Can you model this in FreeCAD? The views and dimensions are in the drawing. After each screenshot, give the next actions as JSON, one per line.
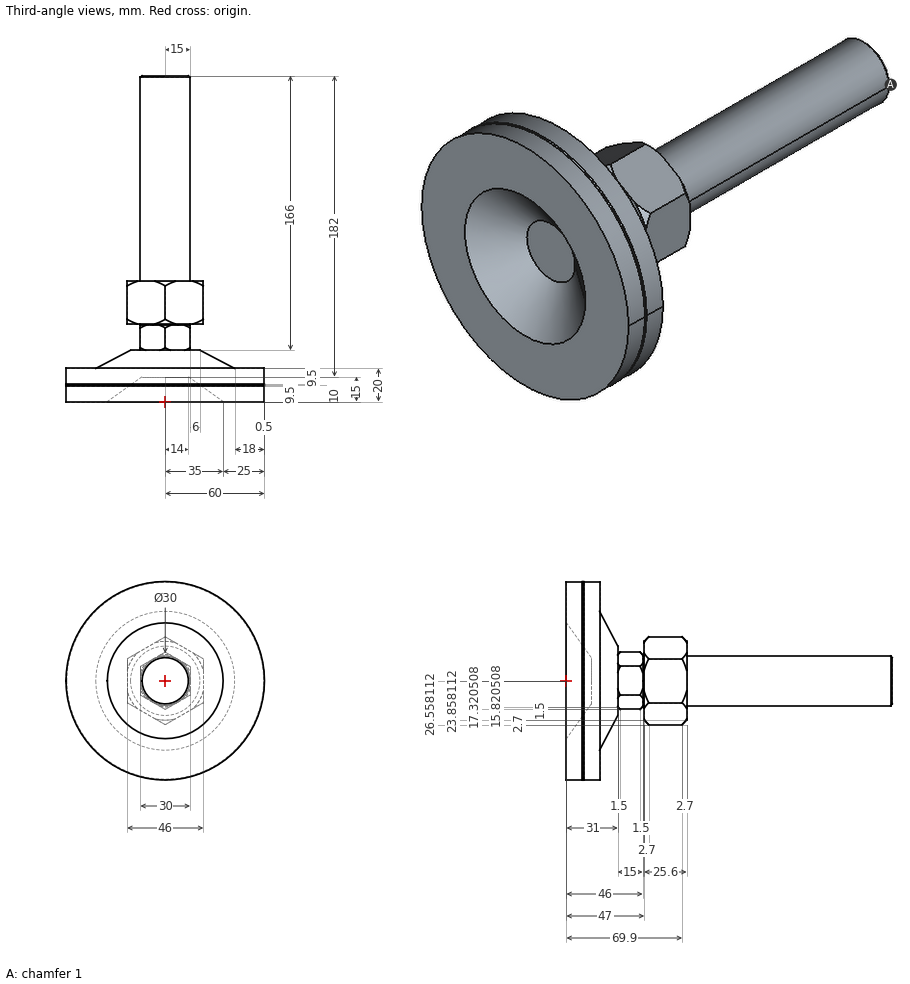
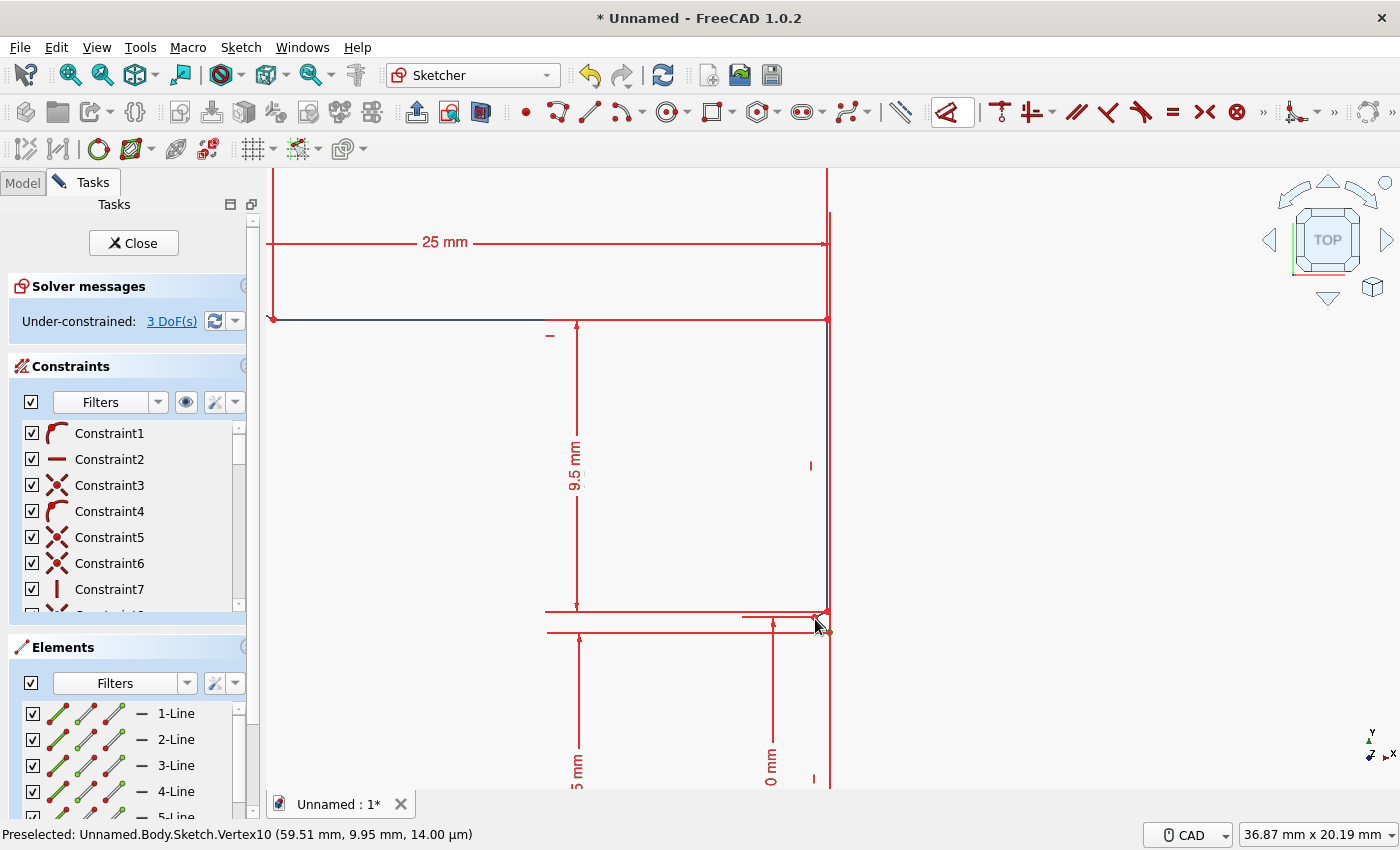
{"action": "left_click", "coordinate": [827, 612]}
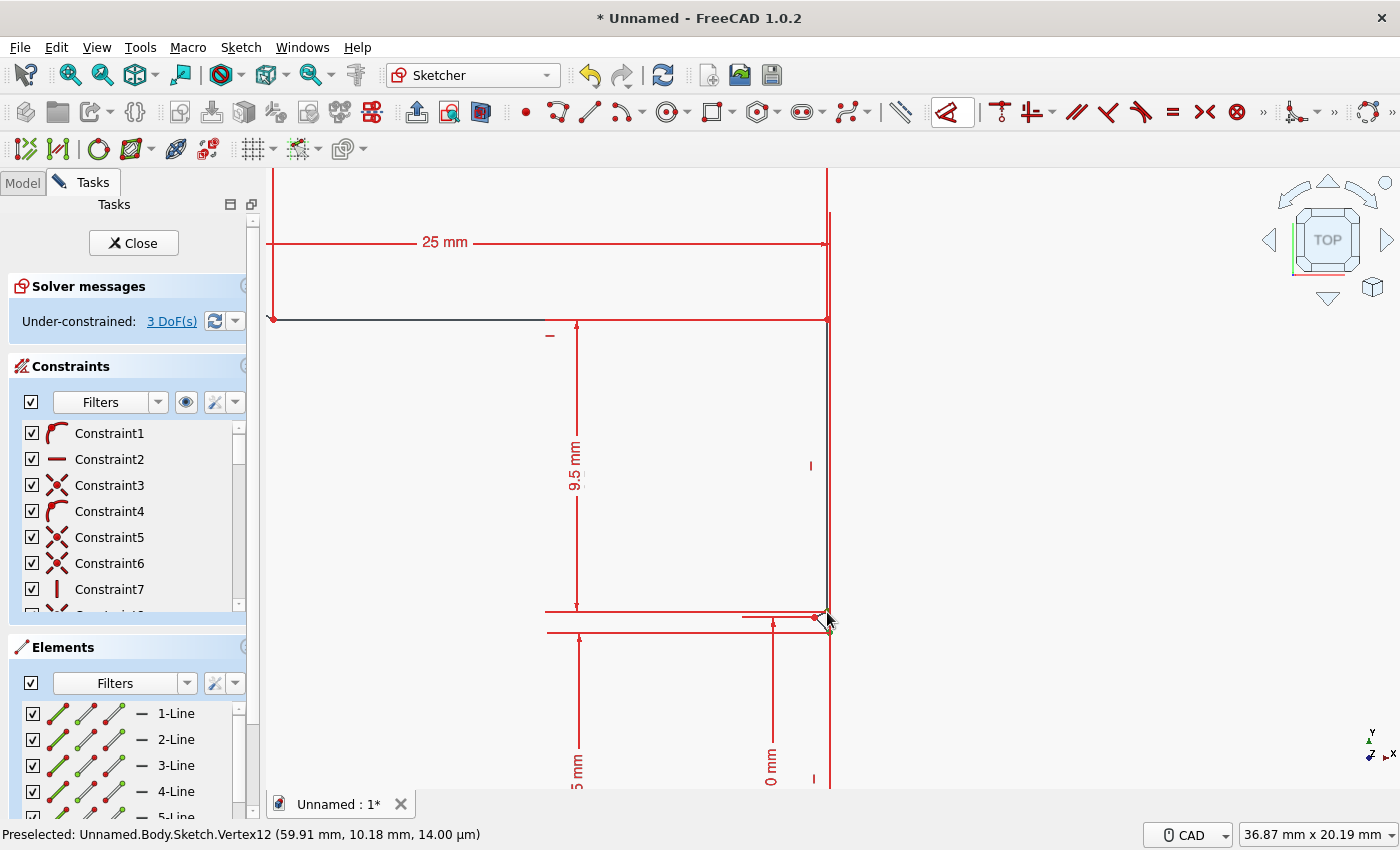
{"action": "key", "text": "l"}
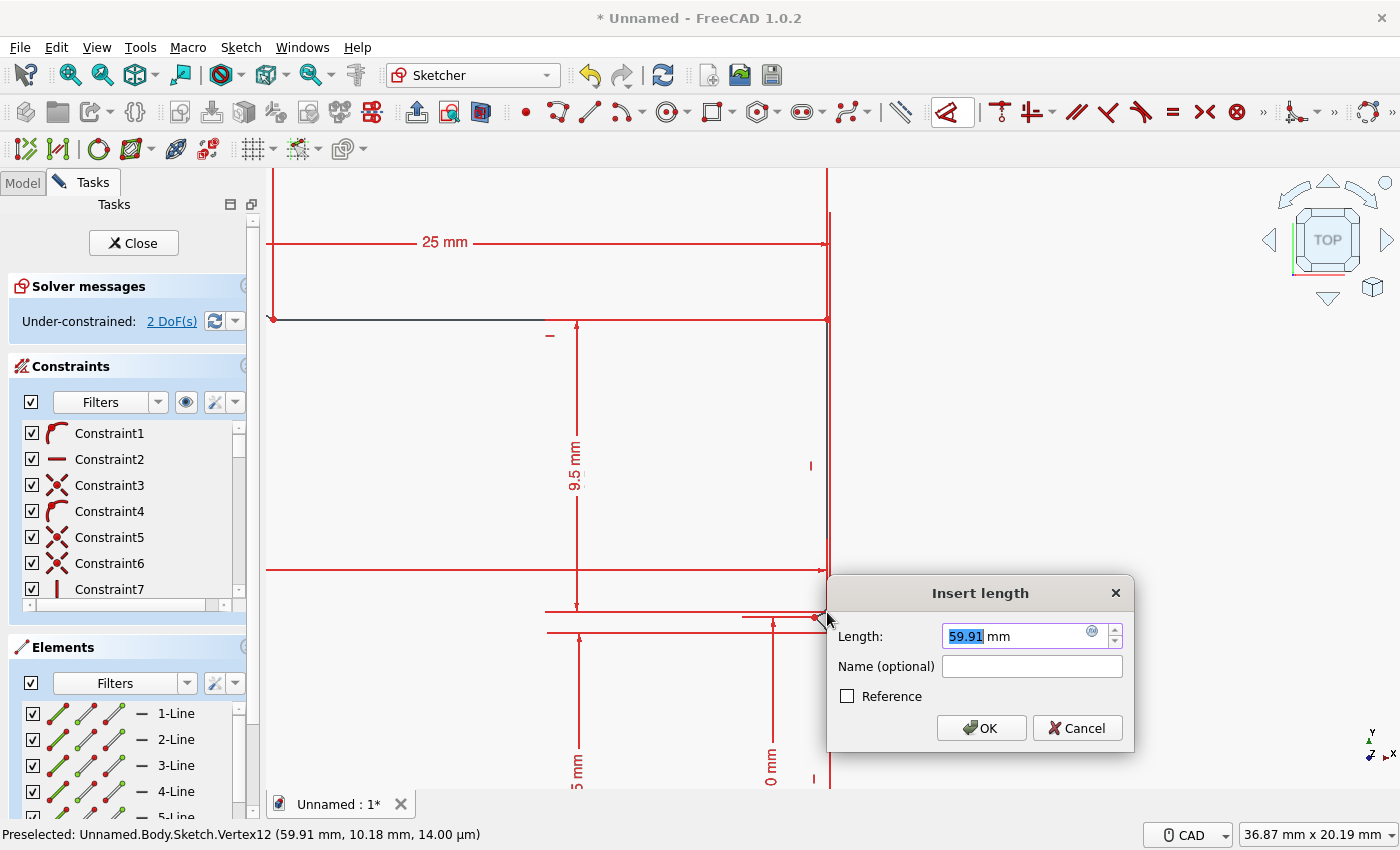
{"action": "type", "text": "60"}
{"action": "key", "text": "Return"}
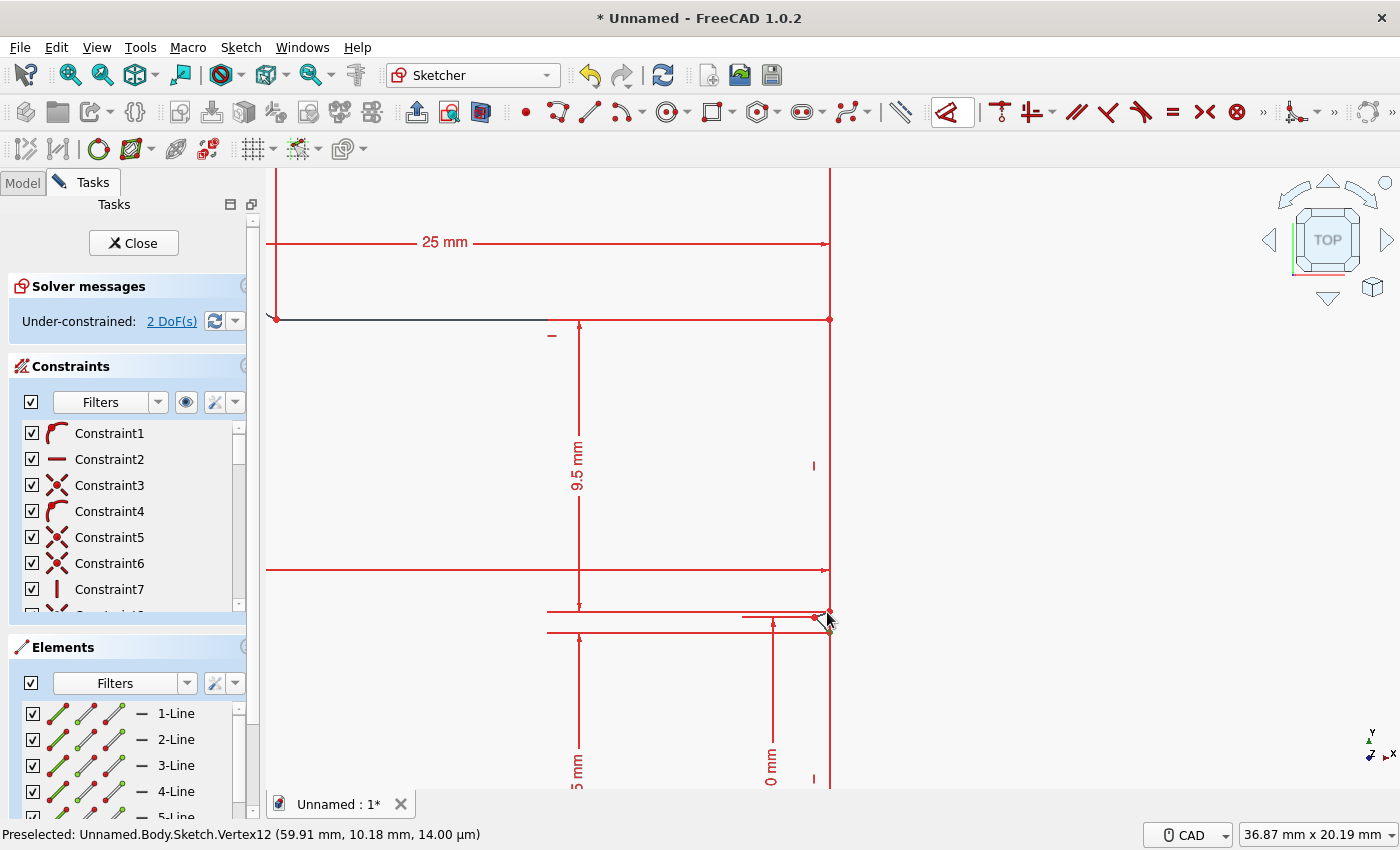
{"action": "scroll", "coordinate": [820, 646], "scroll_direction": "down", "scroll_amount": 14}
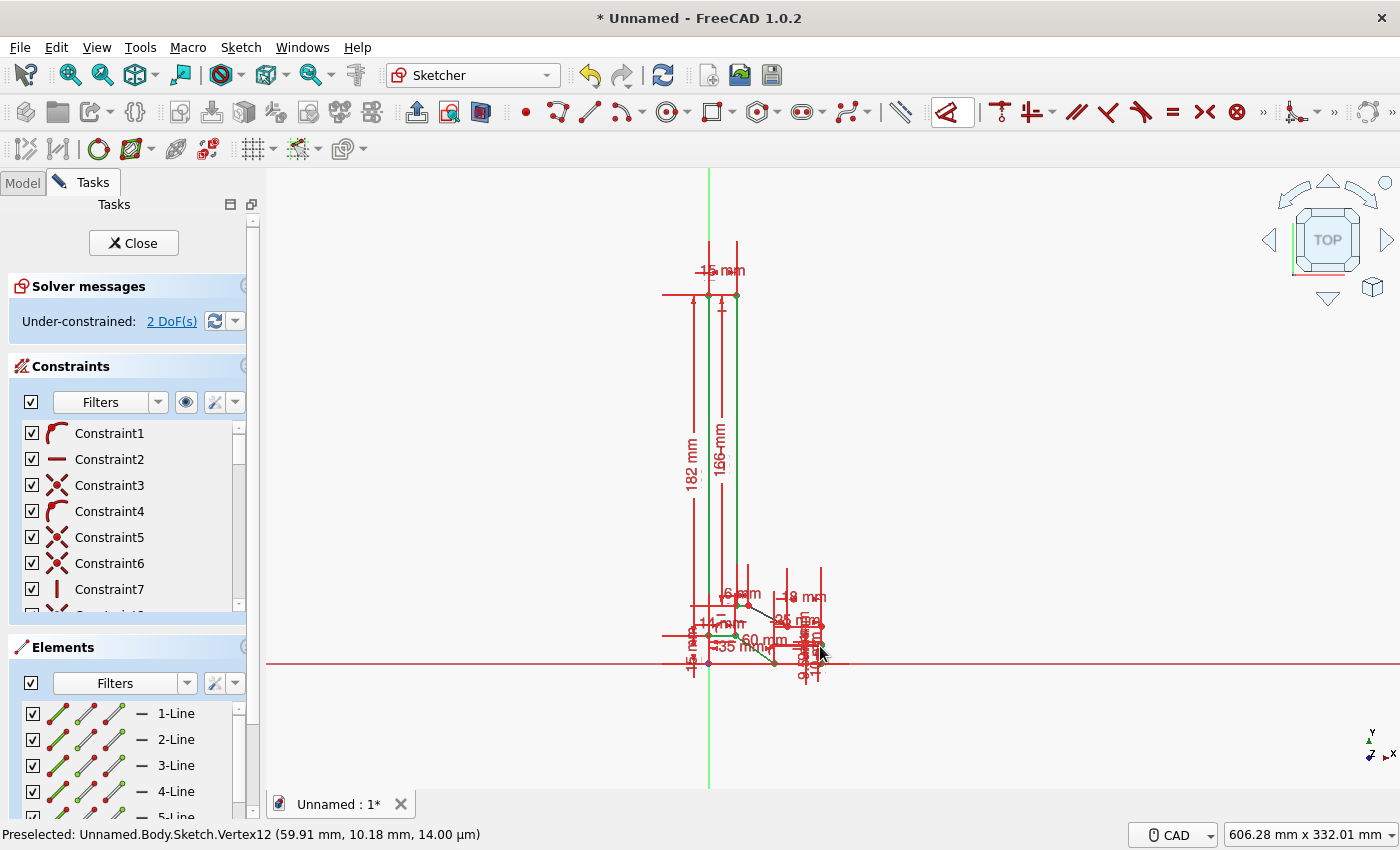
{"action": "left_click", "coordinate": [821, 627]}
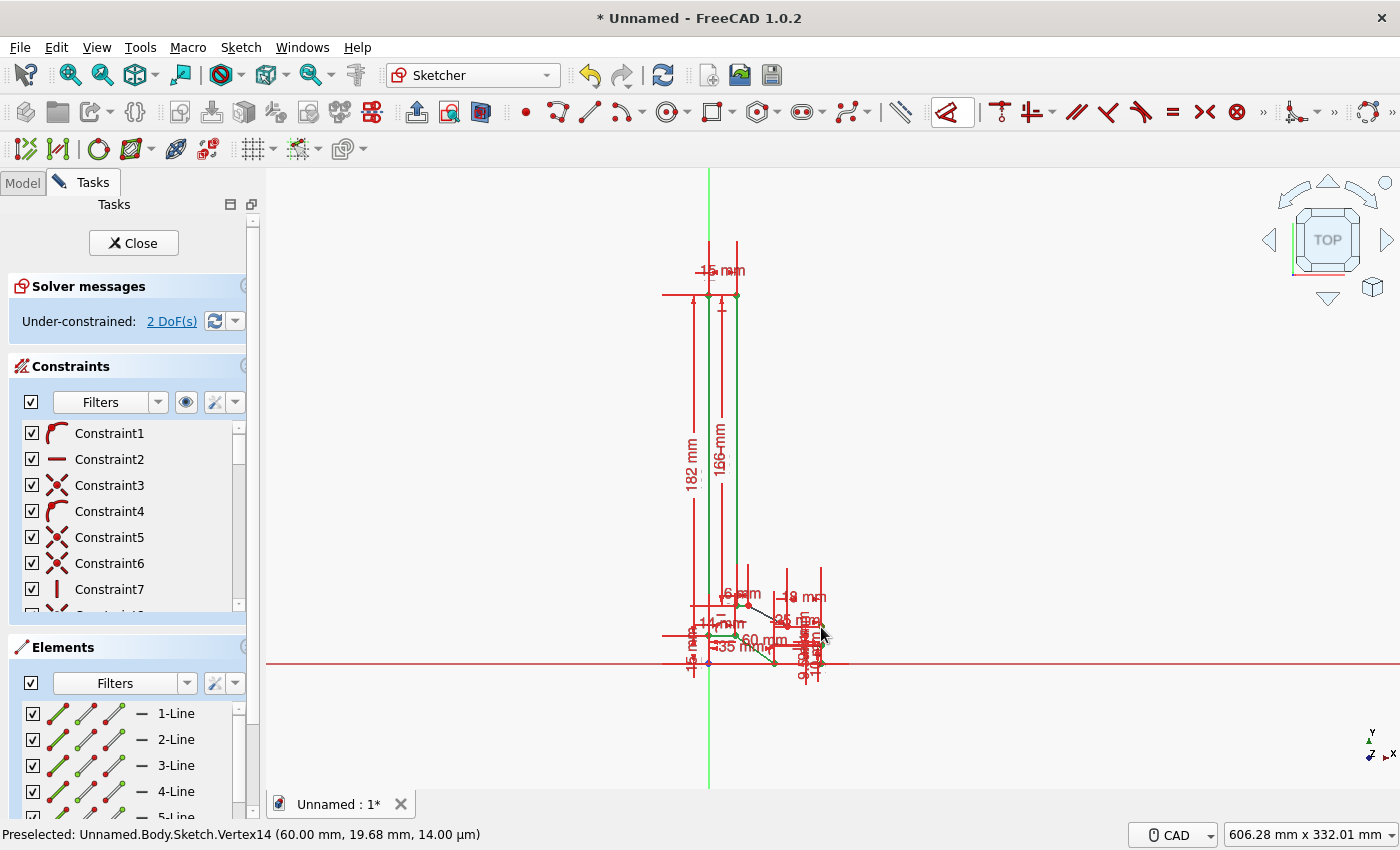
{"action": "key", "text": "i"}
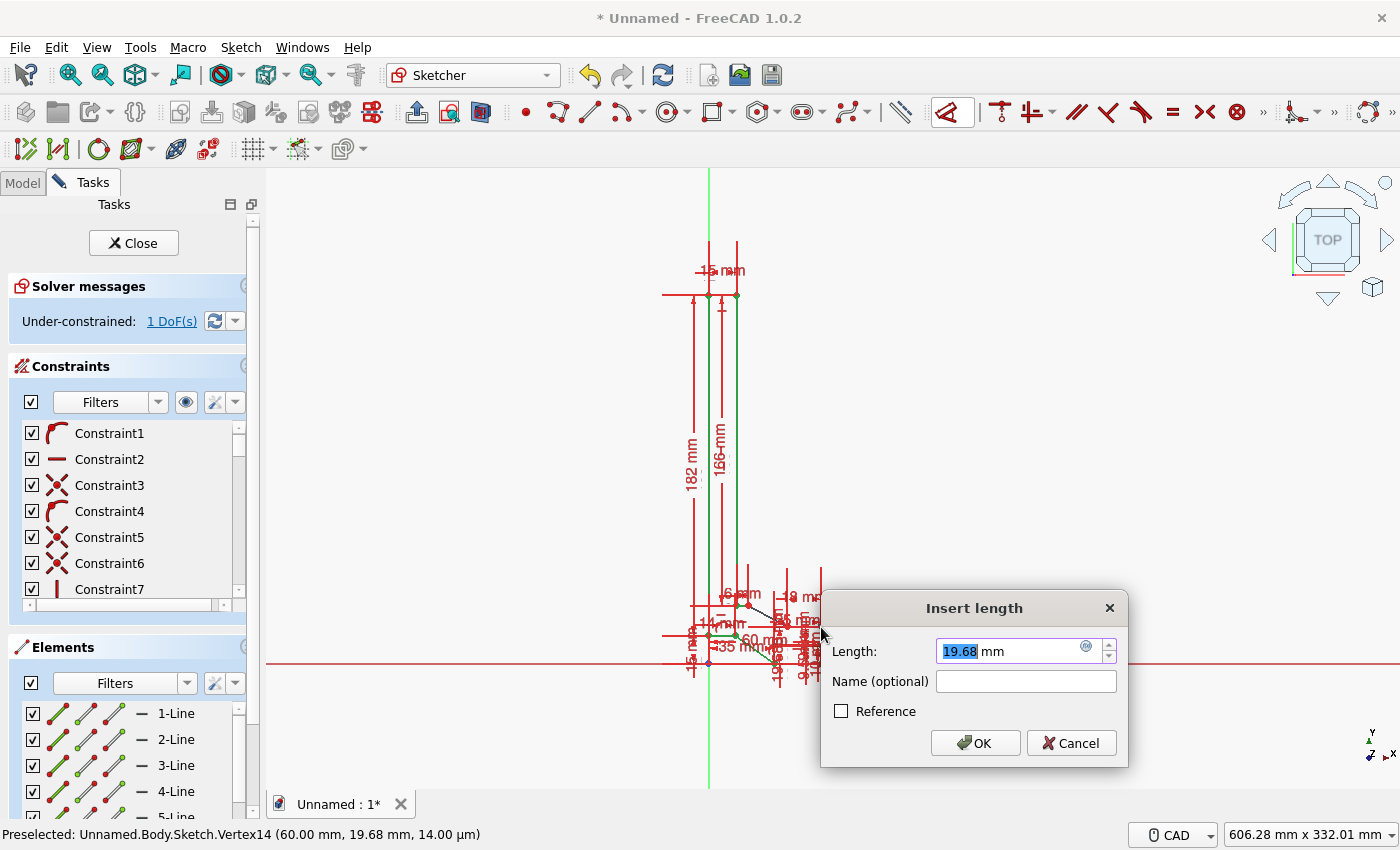
{"action": "type", "text": "20"}
{"action": "key", "text": "Return"}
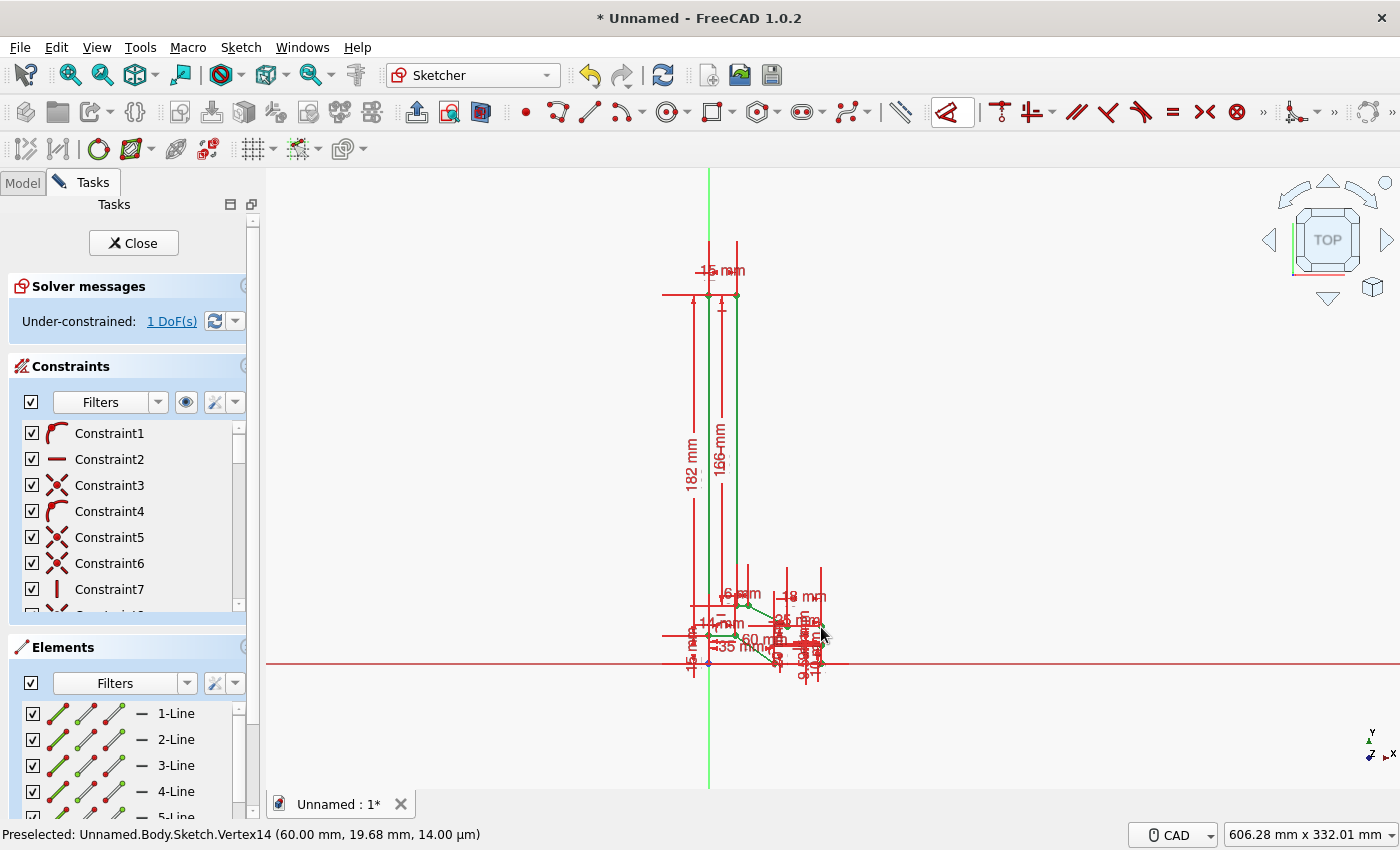
{"action": "scroll", "coordinate": [821, 645], "scroll_direction": "up", "scroll_amount": 19}